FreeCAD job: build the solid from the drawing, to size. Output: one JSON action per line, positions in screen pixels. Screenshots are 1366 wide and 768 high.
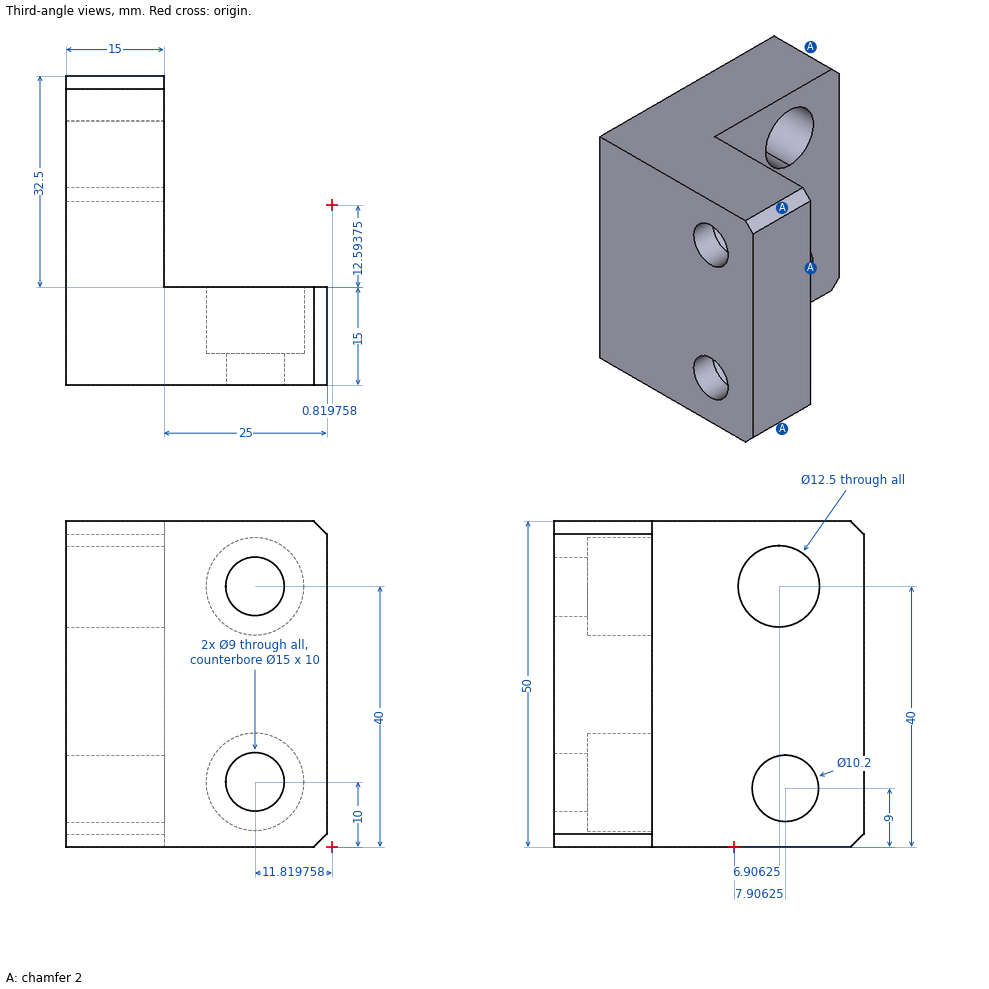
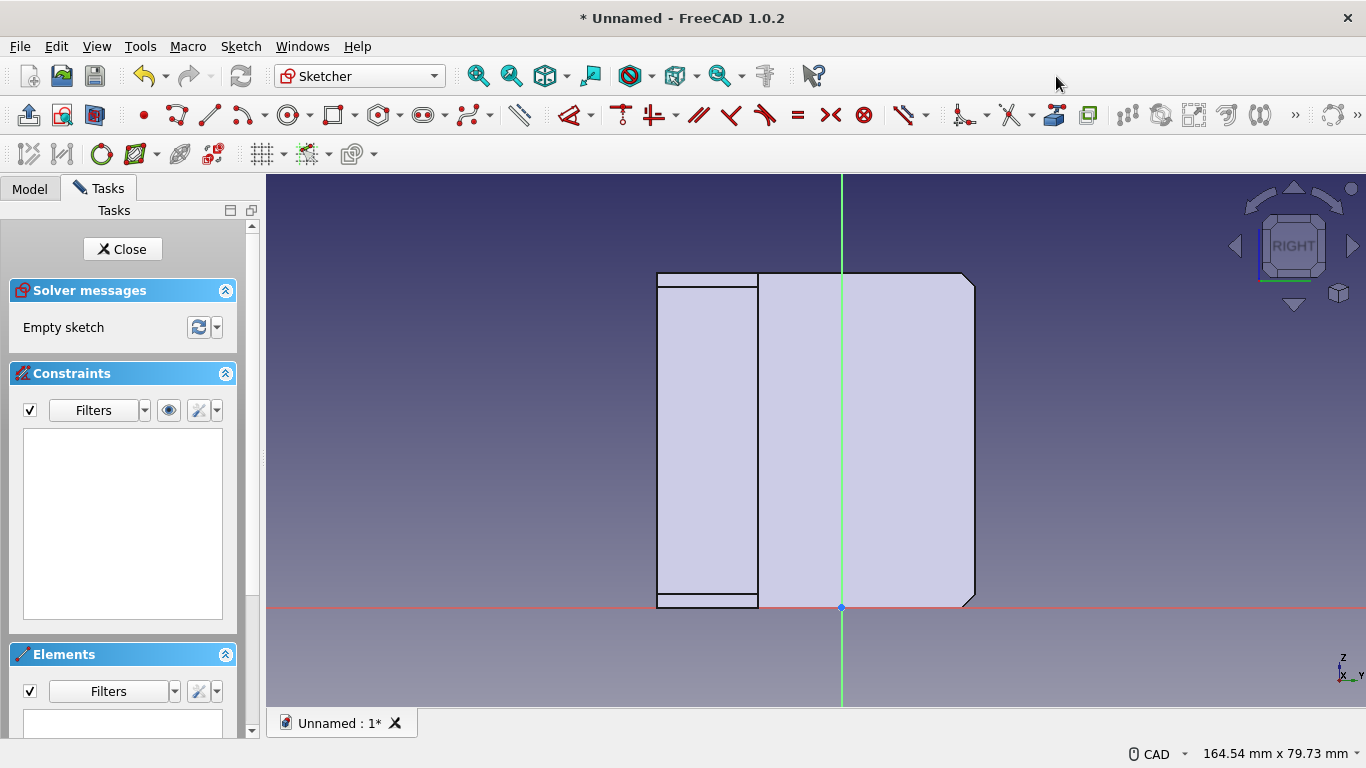
{"action": "left_click", "coordinate": [95, 116]}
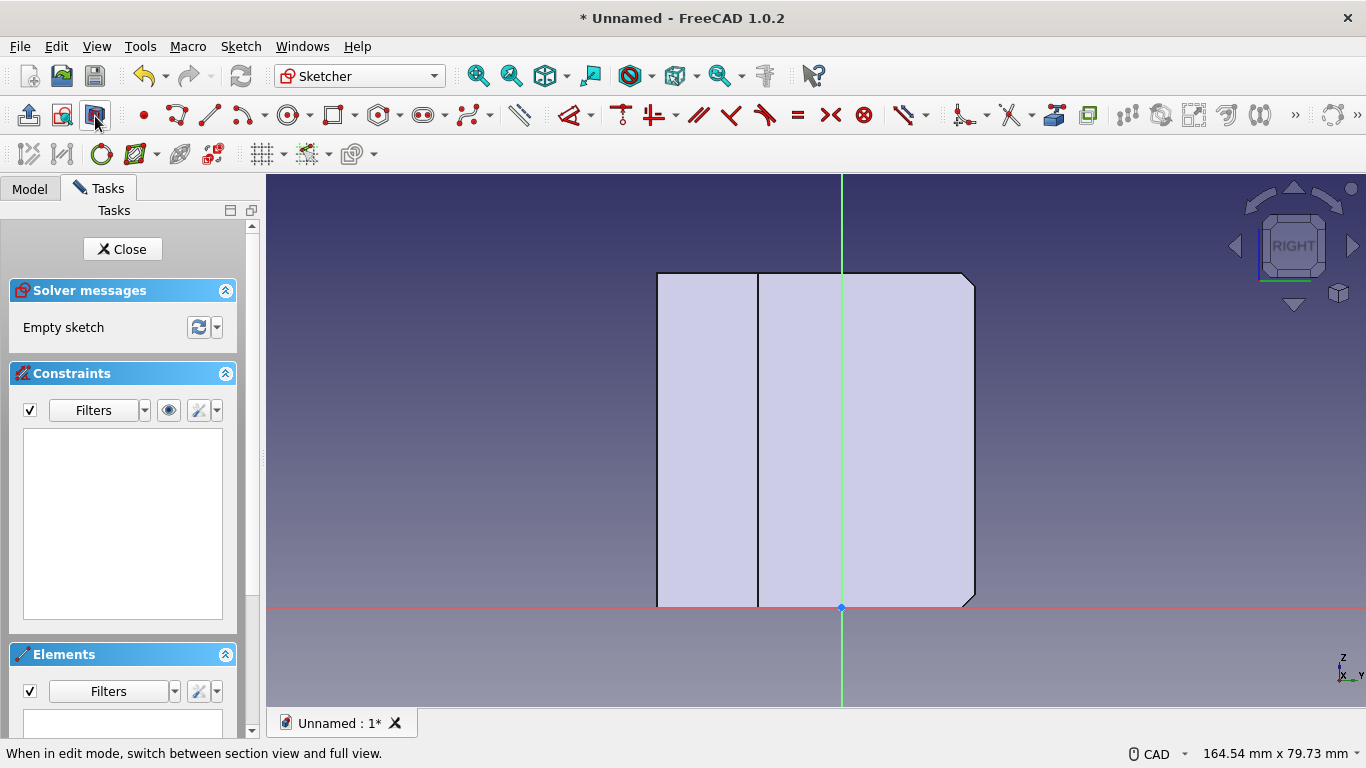
{"action": "scroll", "coordinate": [934, 307], "scroll_direction": "up", "scroll_amount": 7}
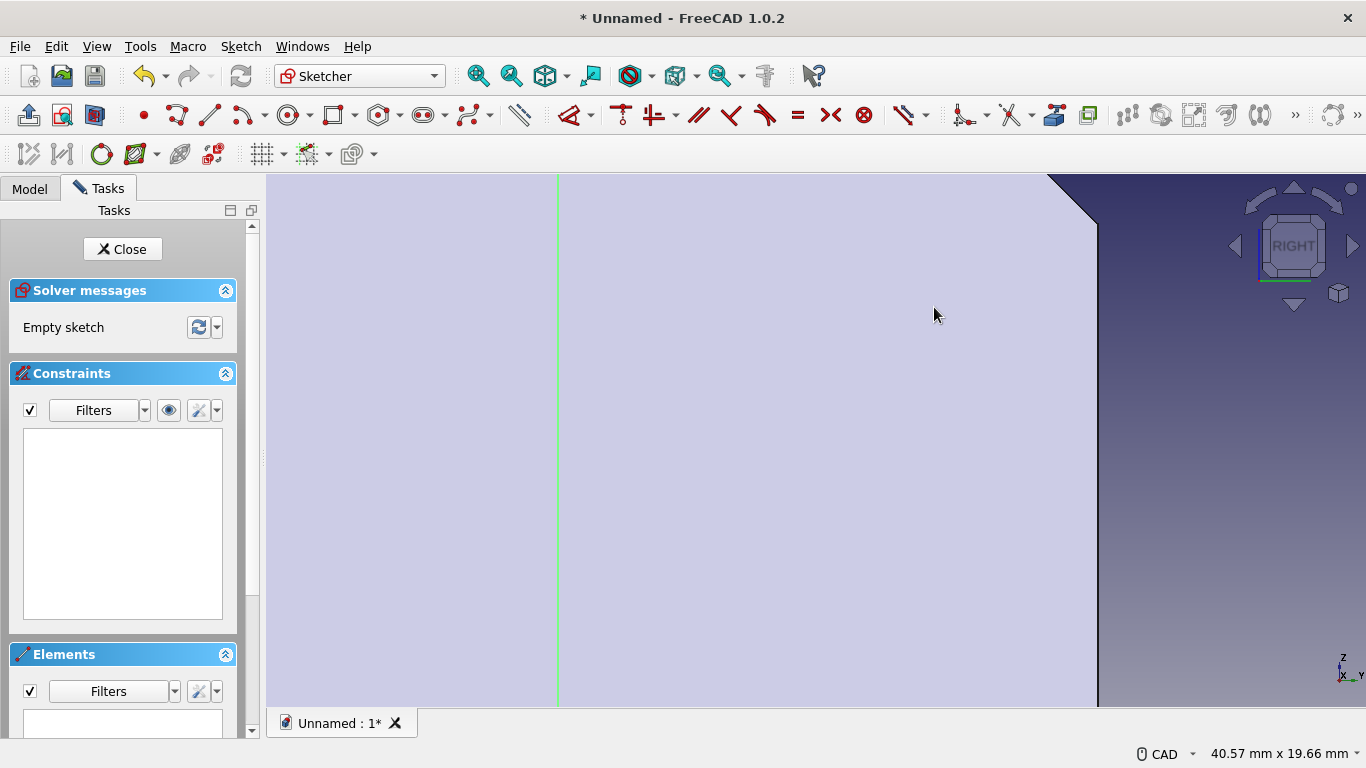
{"action": "left_click", "coordinate": [288, 116]}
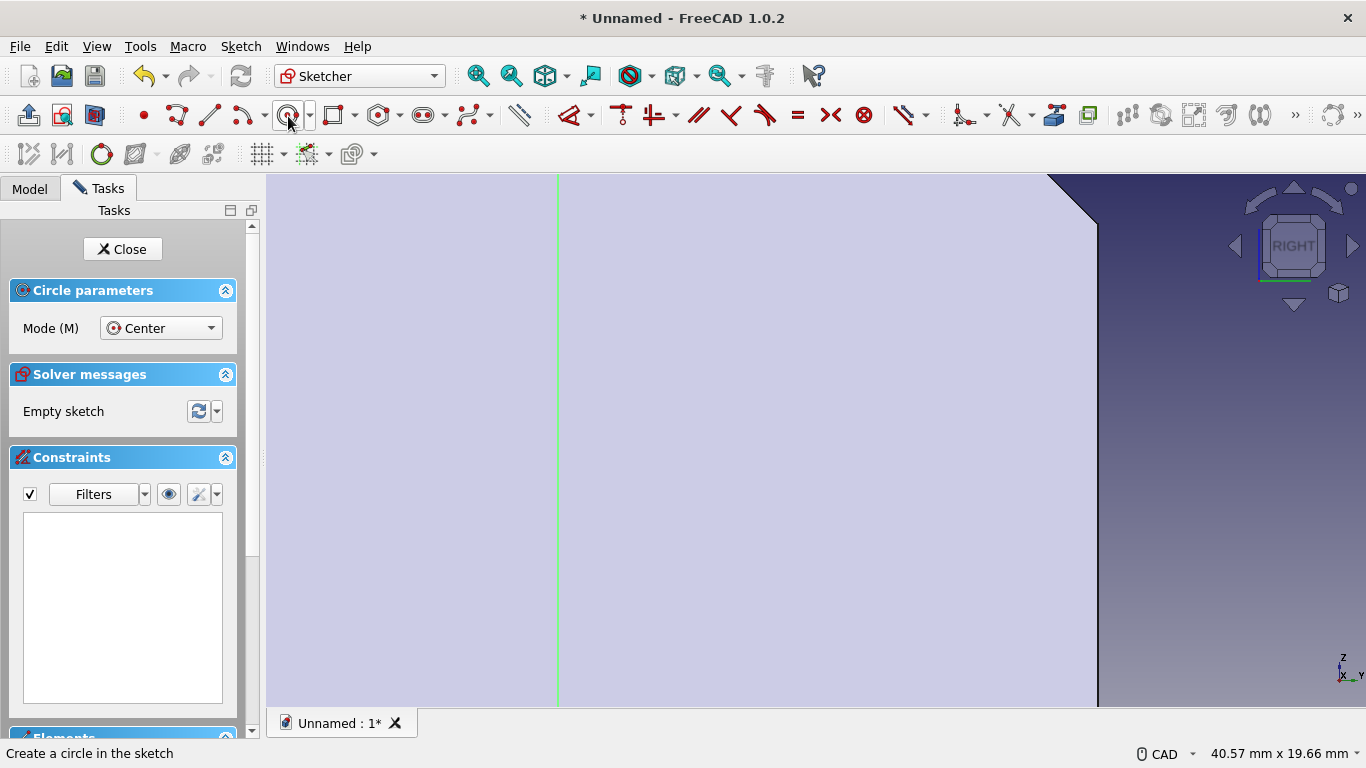
{"action": "left_click", "coordinate": [745, 441]}
{"action": "left_click", "coordinate": [865, 321]}
{"action": "key", "text": "Escape"}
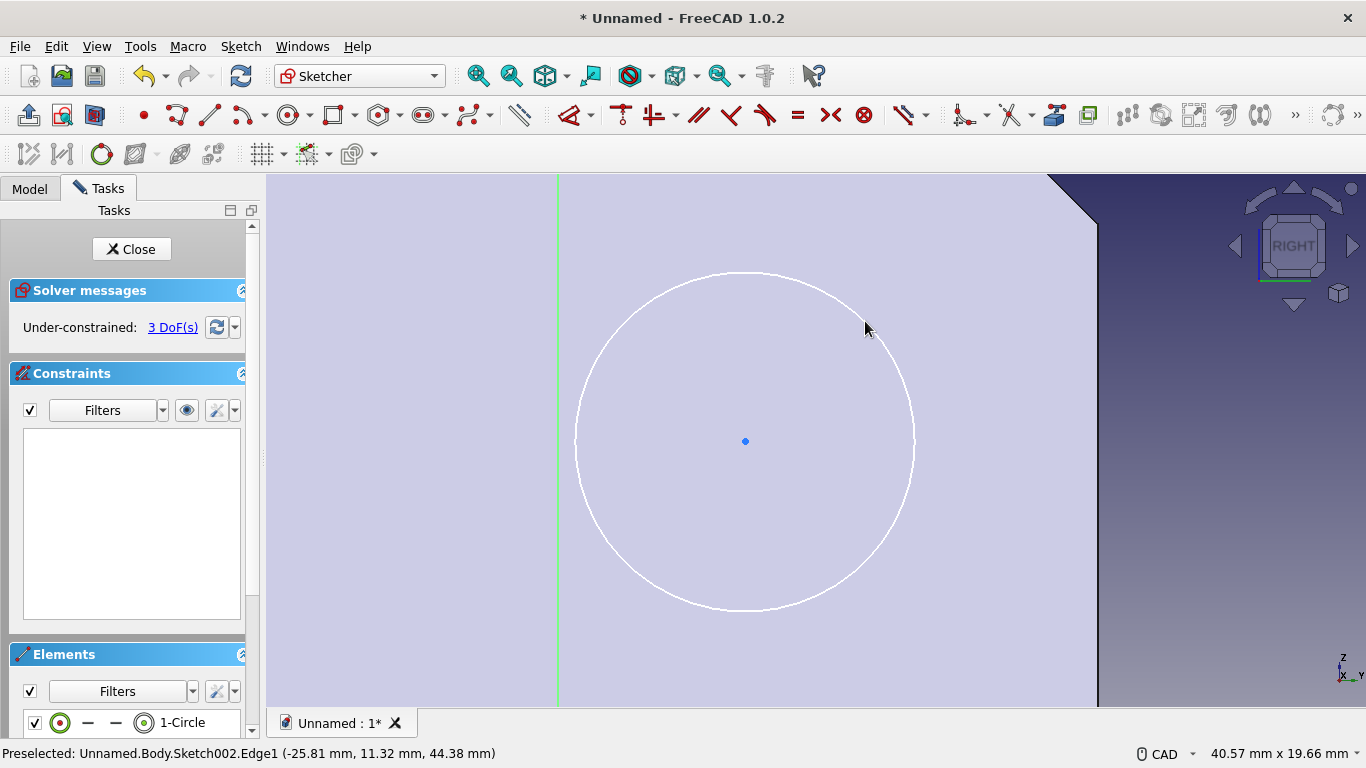
{"action": "left_click", "coordinate": [568, 116]}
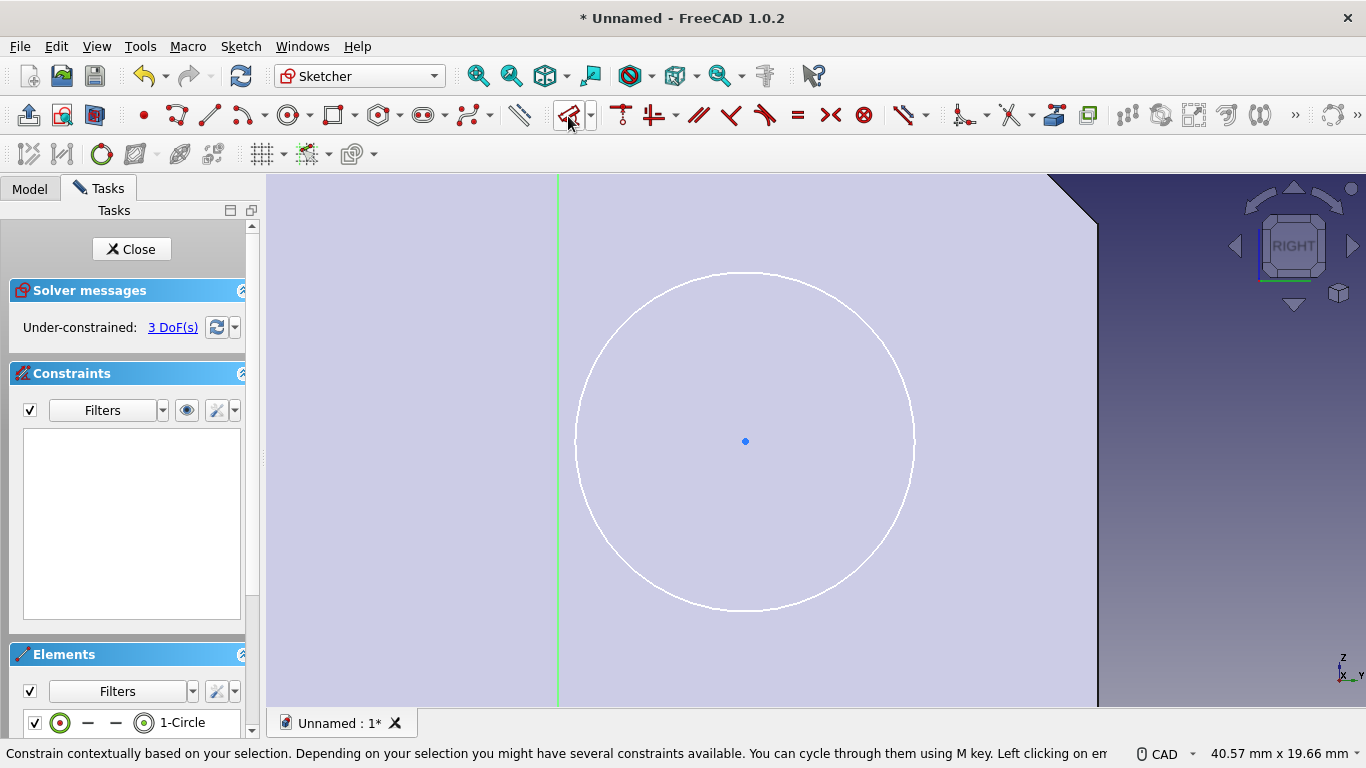
{"action": "left_click", "coordinate": [865, 322]}
{"action": "left_click", "coordinate": [888, 299]}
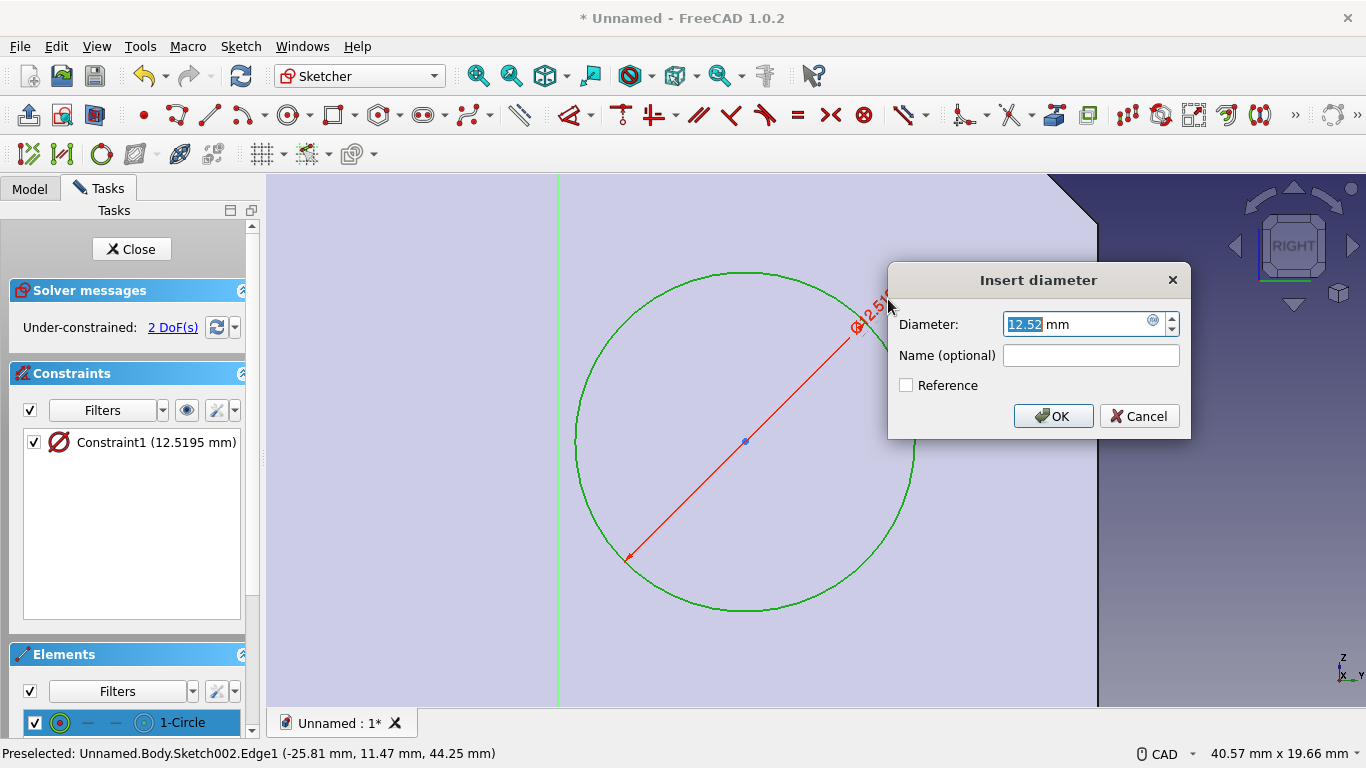
{"action": "type", "text": "12.5"}
{"action": "key", "text": "Return"}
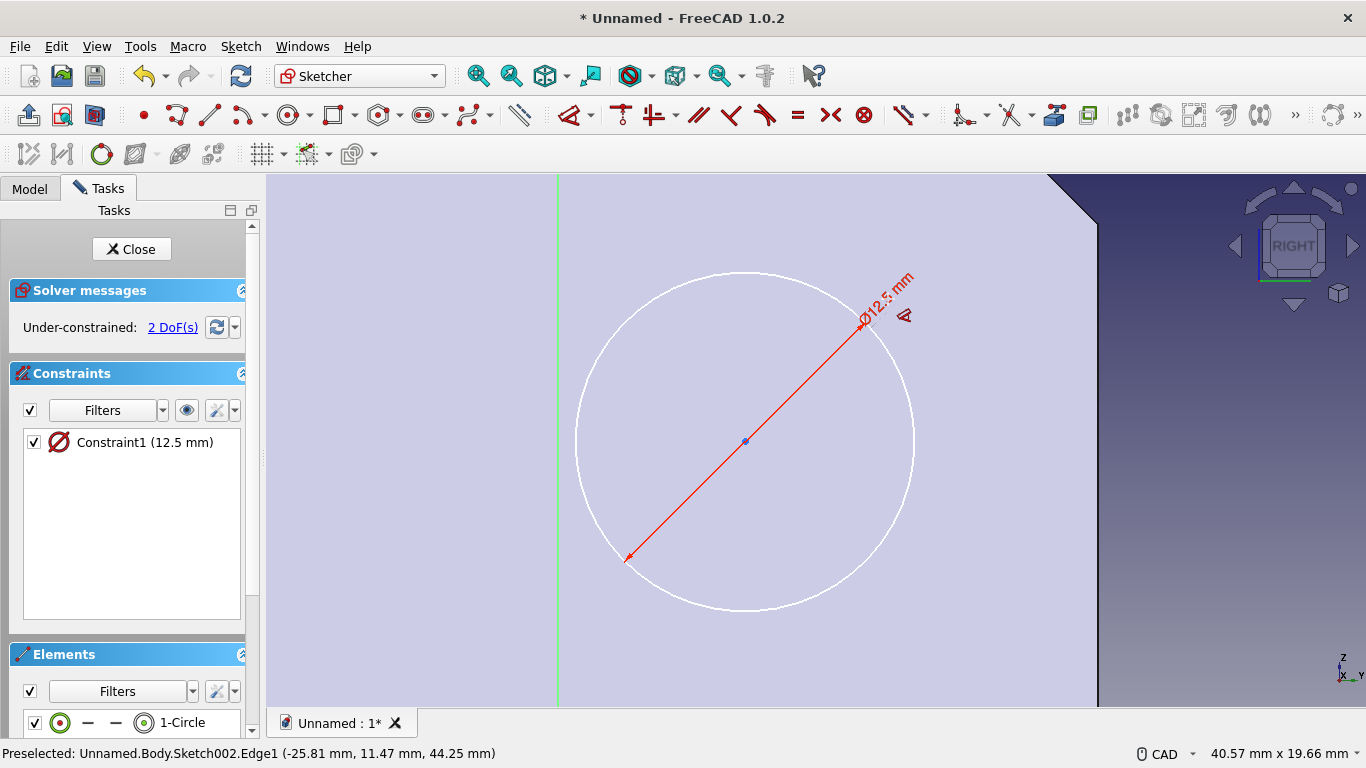
{"action": "left_click", "coordinate": [745, 442]}
{"action": "left_click", "coordinate": [524, 560]}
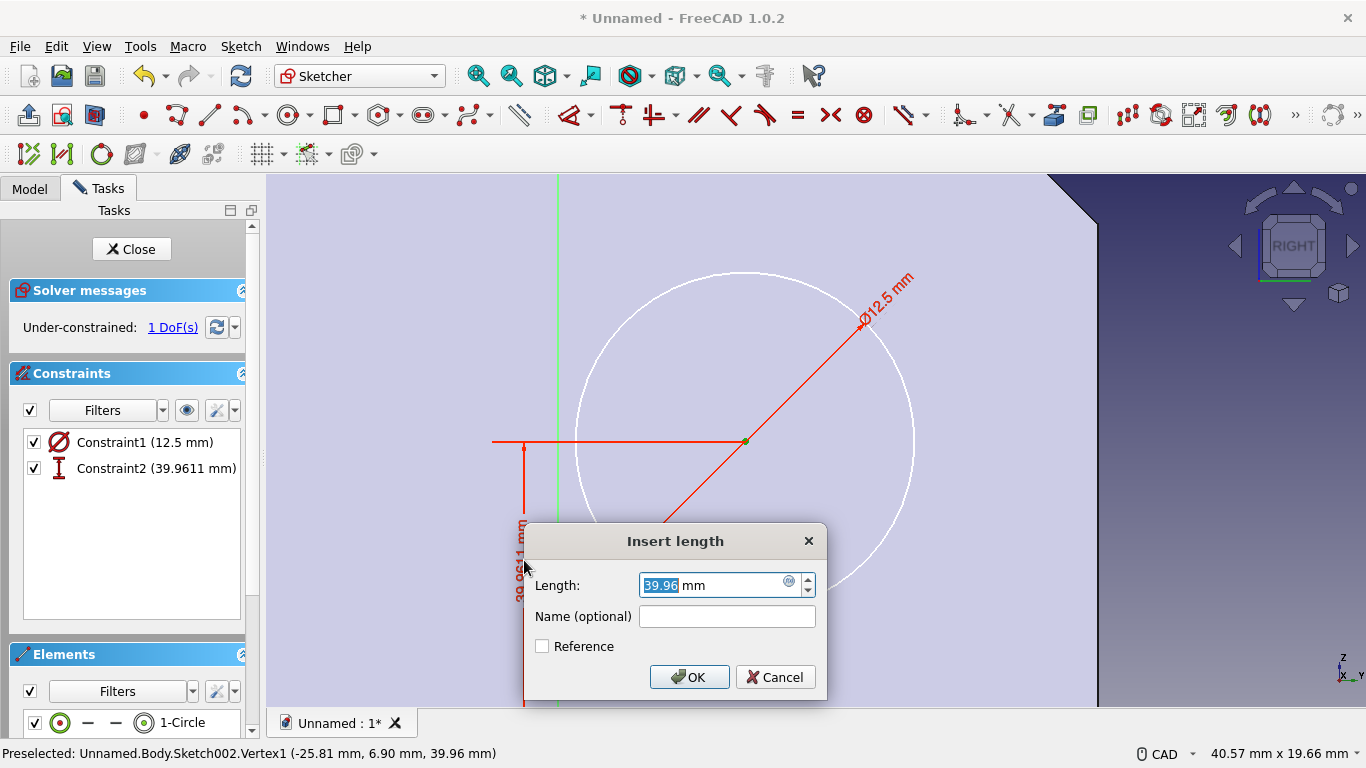
{"action": "type", "text": "40"}
{"action": "key", "text": "Return"}